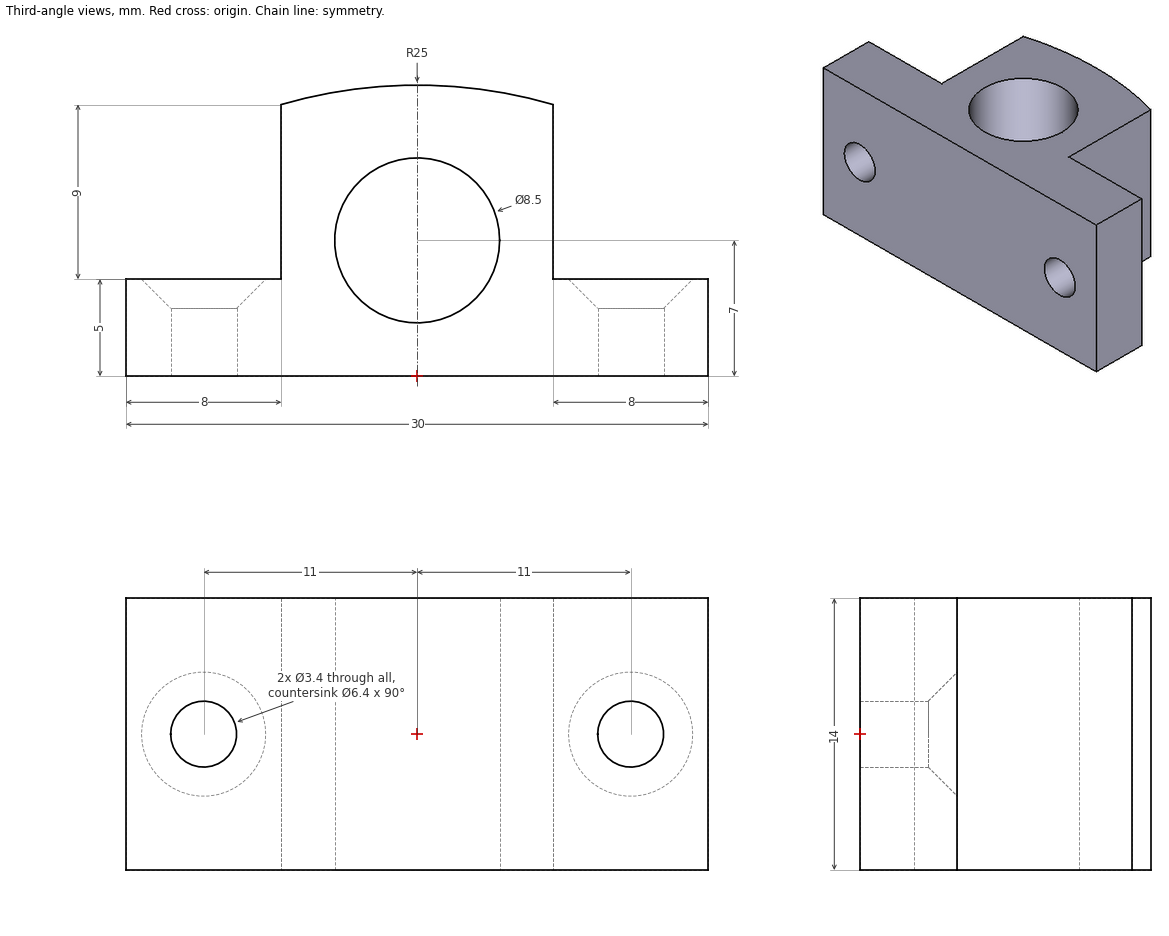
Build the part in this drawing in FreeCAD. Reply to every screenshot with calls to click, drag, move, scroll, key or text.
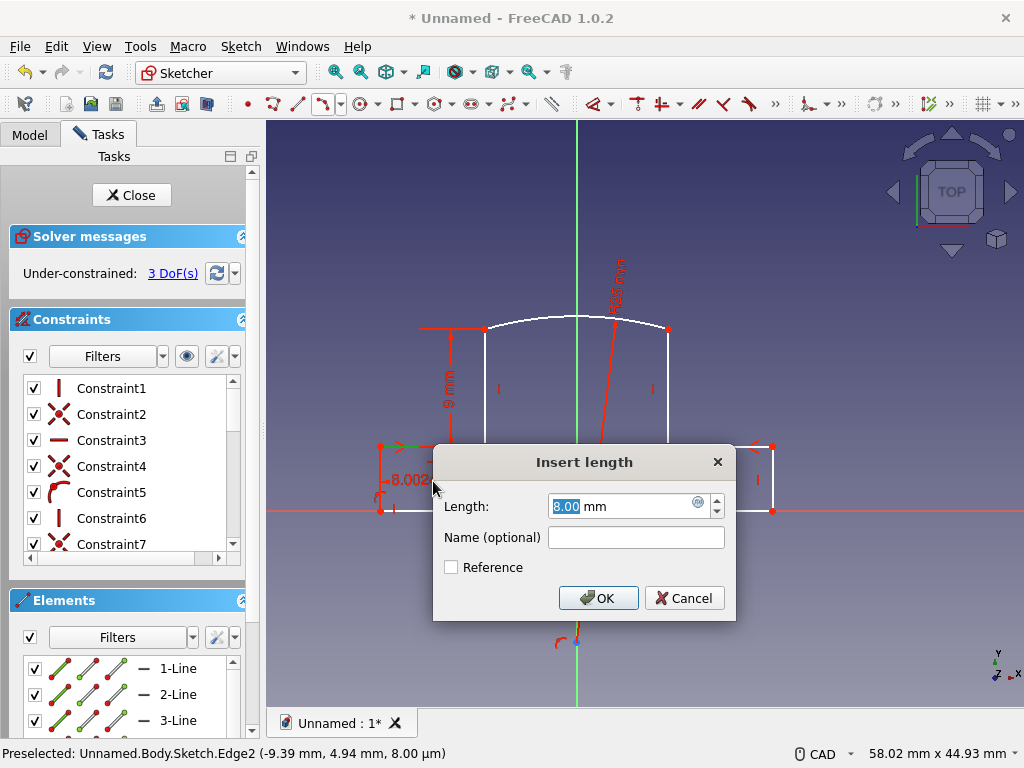
text(8)
key(Return)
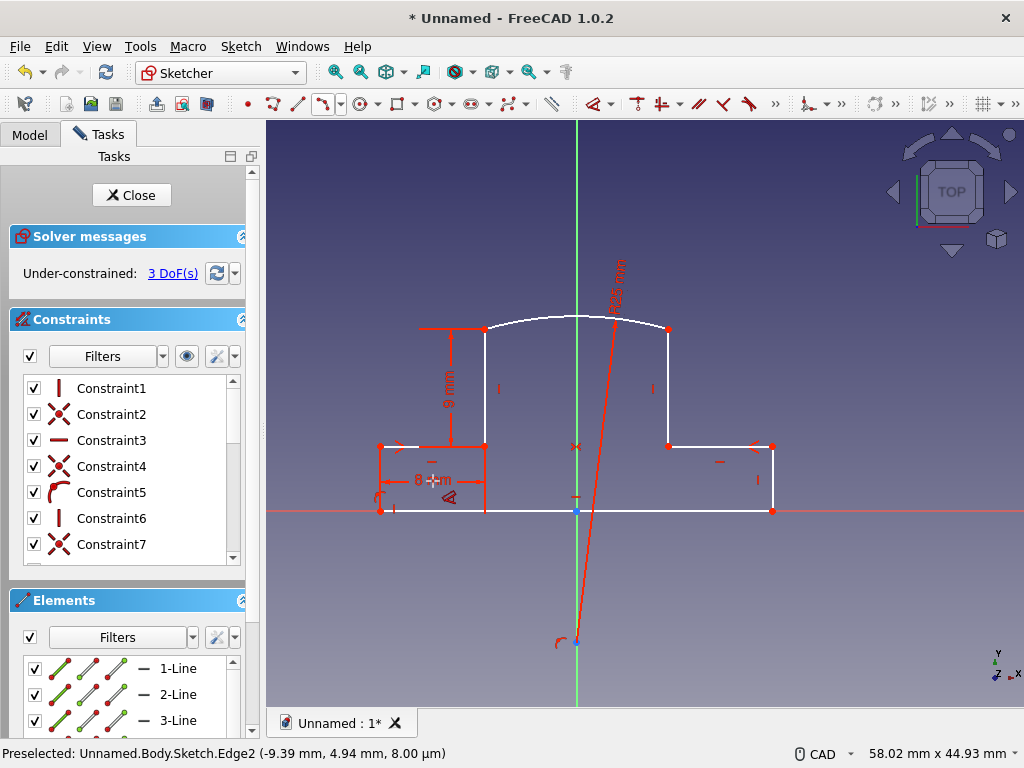
click(380, 466)
click(346, 479)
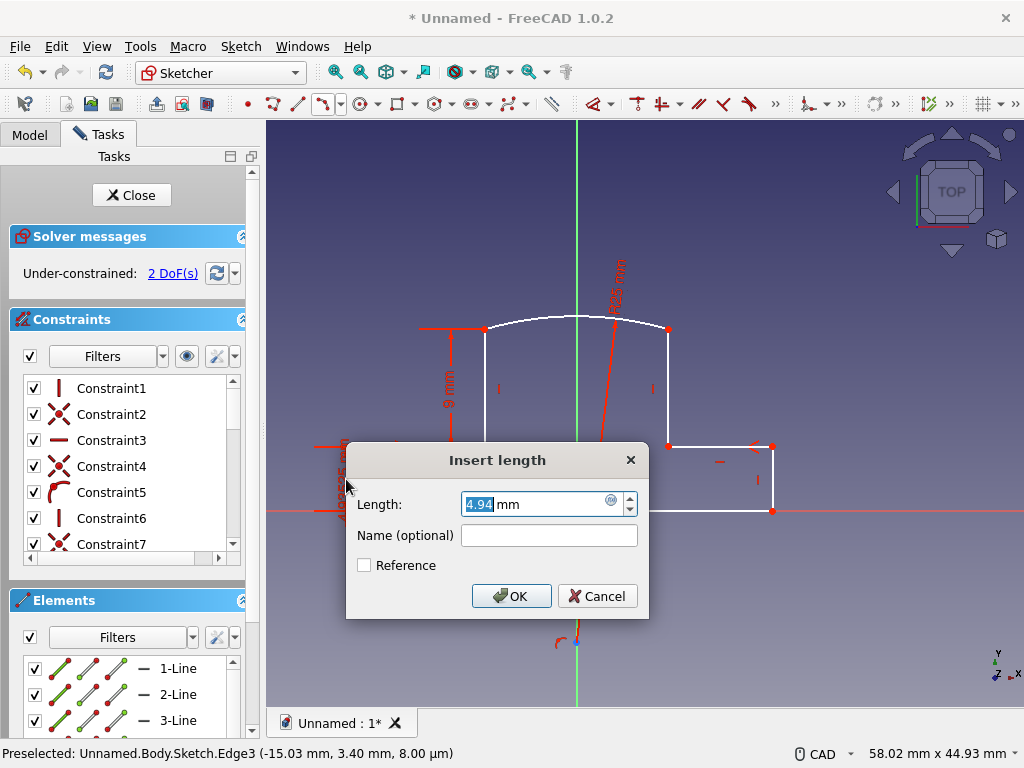
text(5)
key(Return)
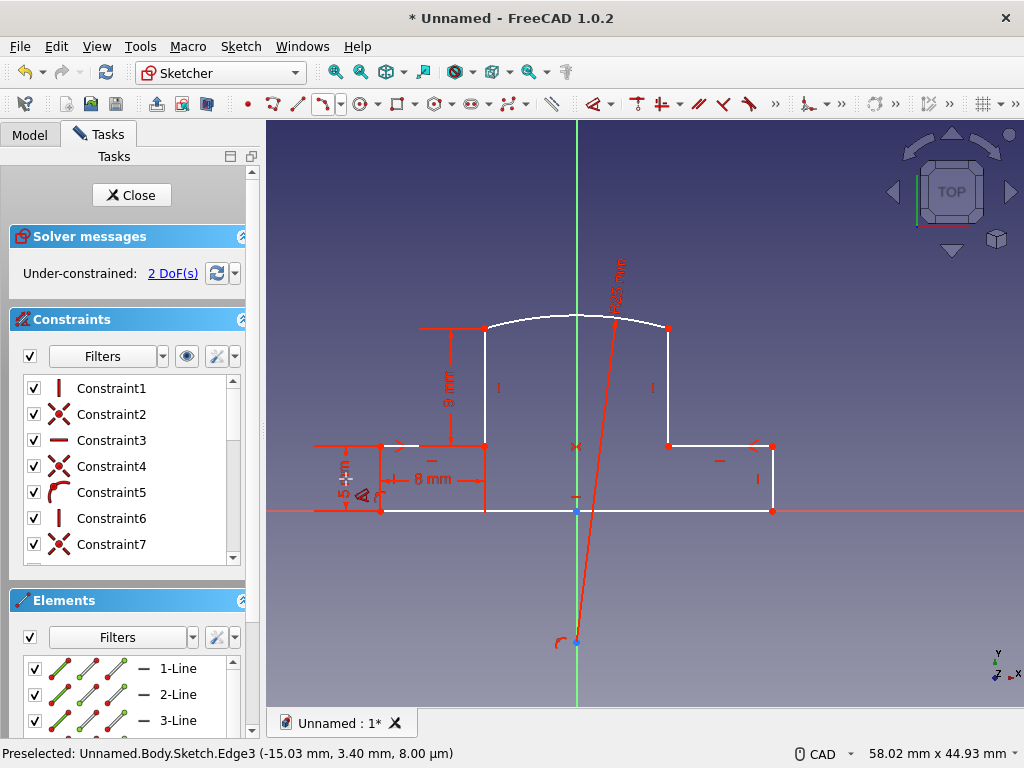
click(742, 446)
click(721, 480)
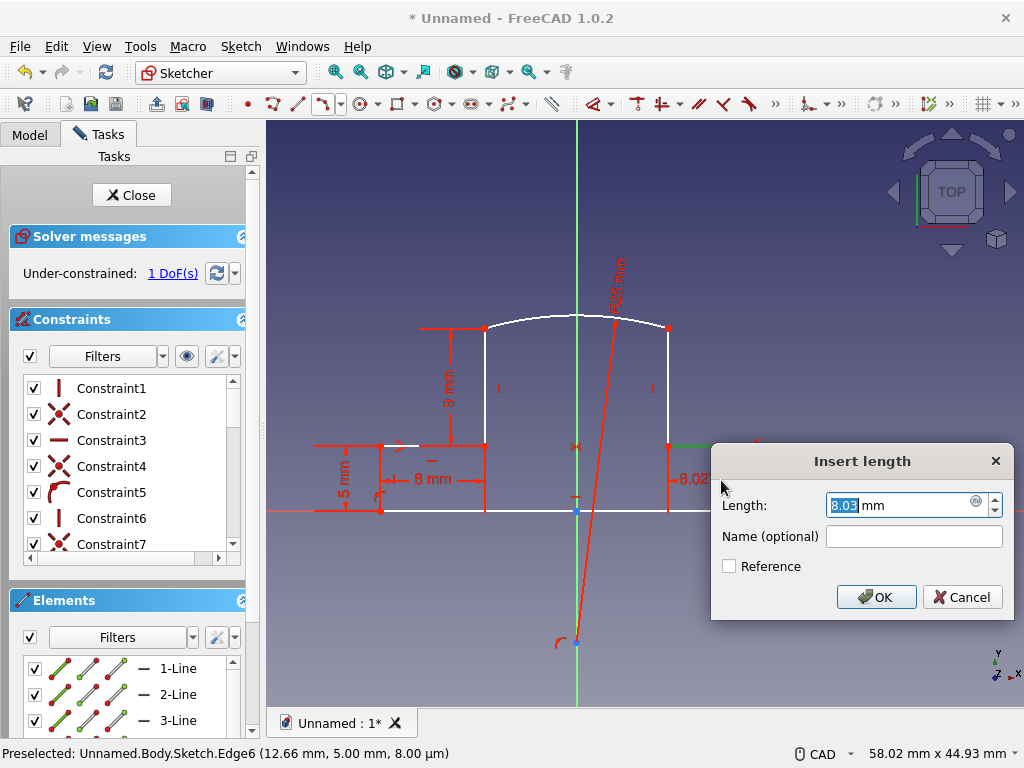
text(8)
key(Return)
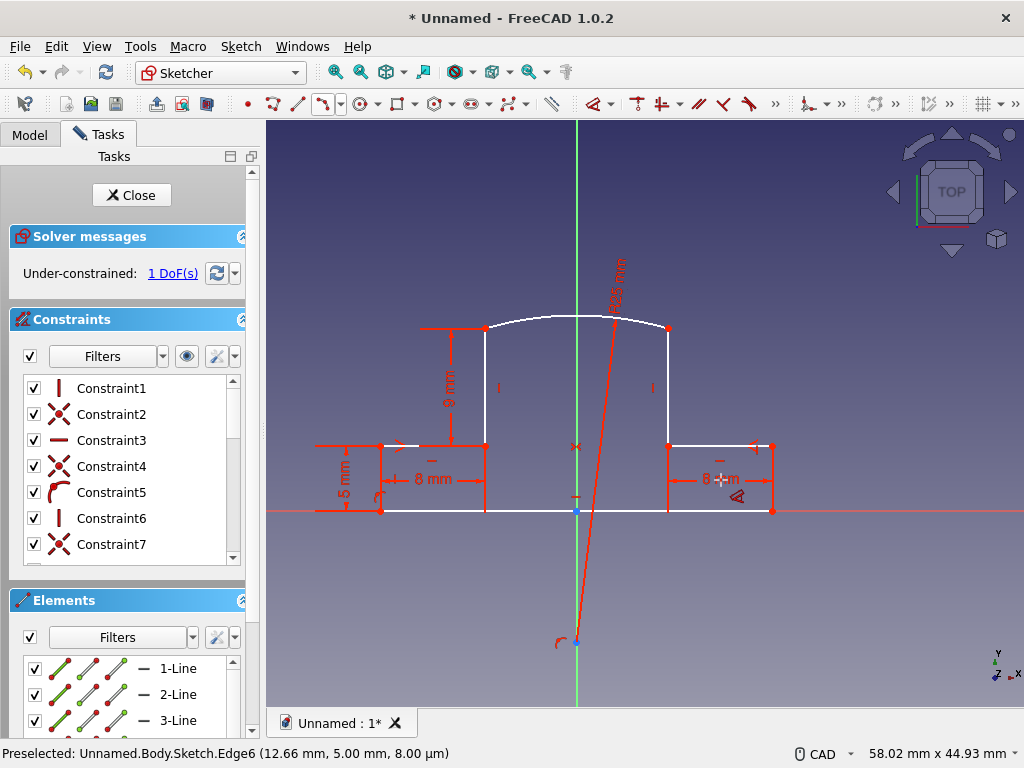
click(498, 511)
click(487, 545)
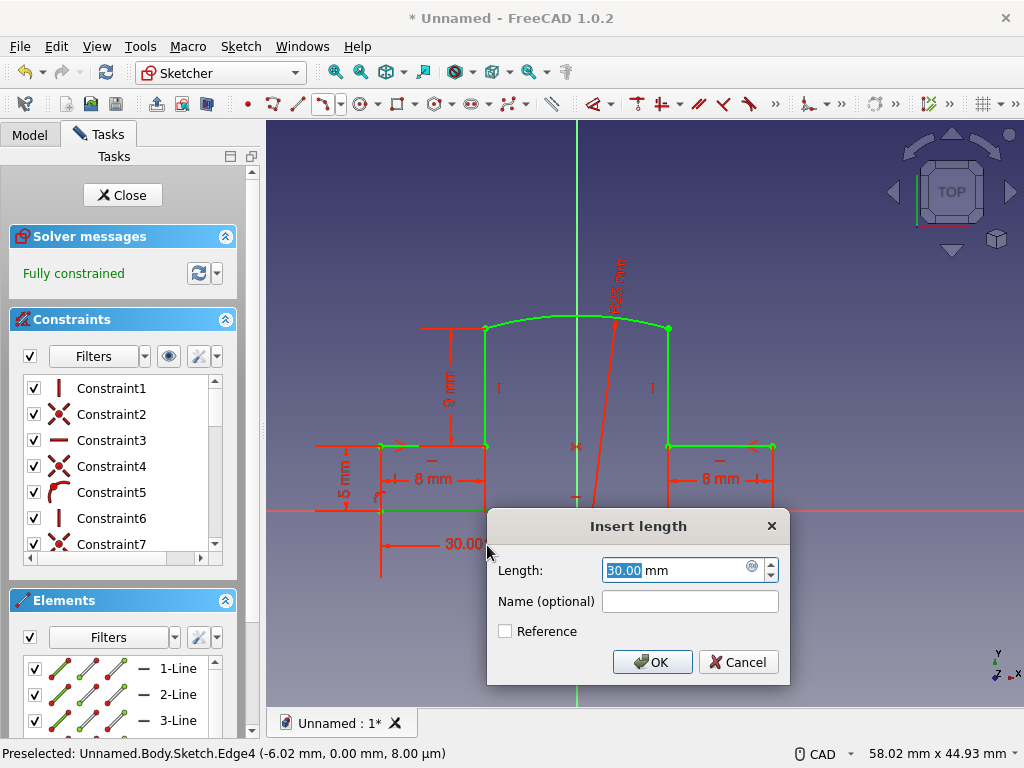
text(30)
key(Return)
key(Escape)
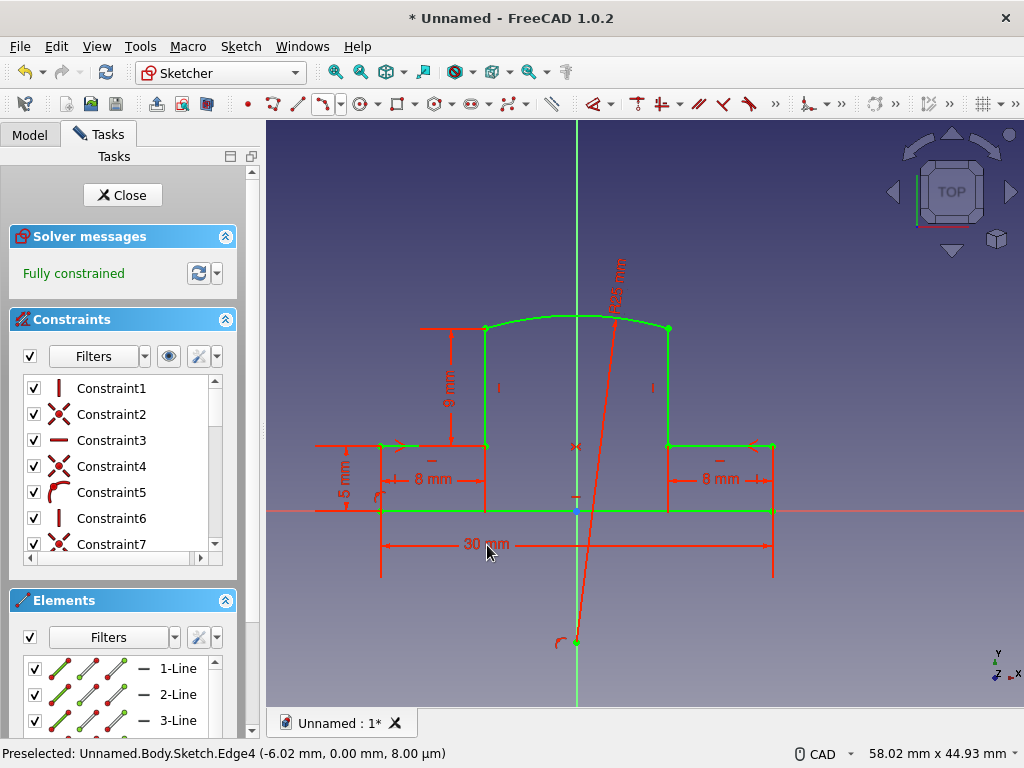
click(123, 195)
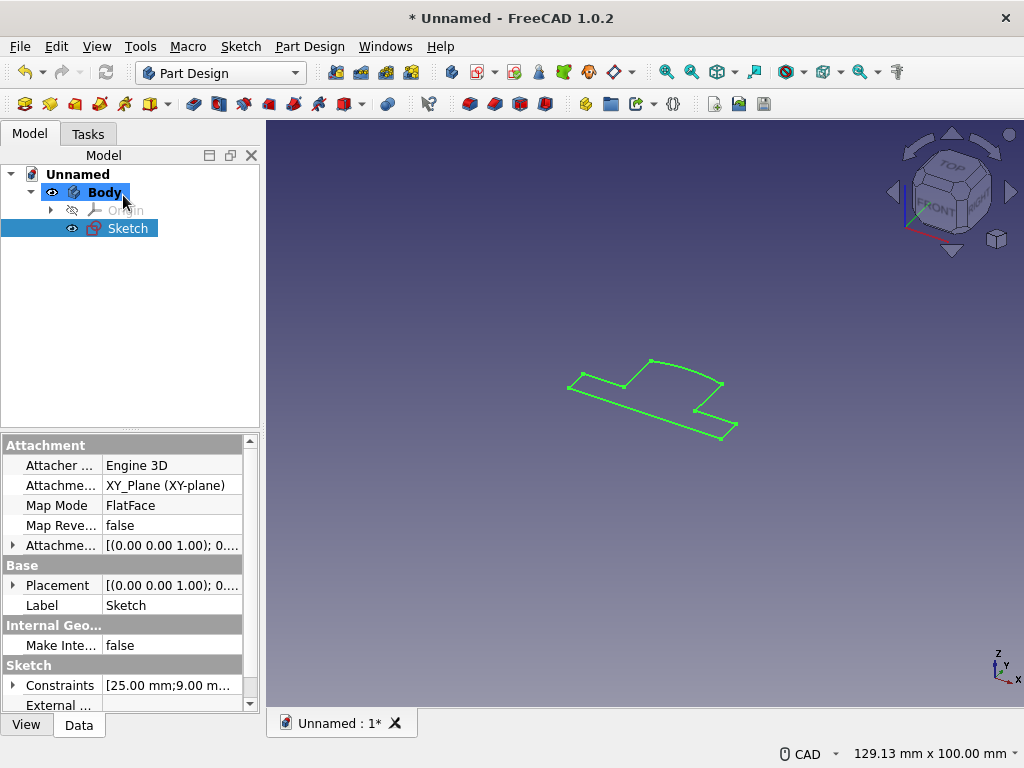
click(25, 104)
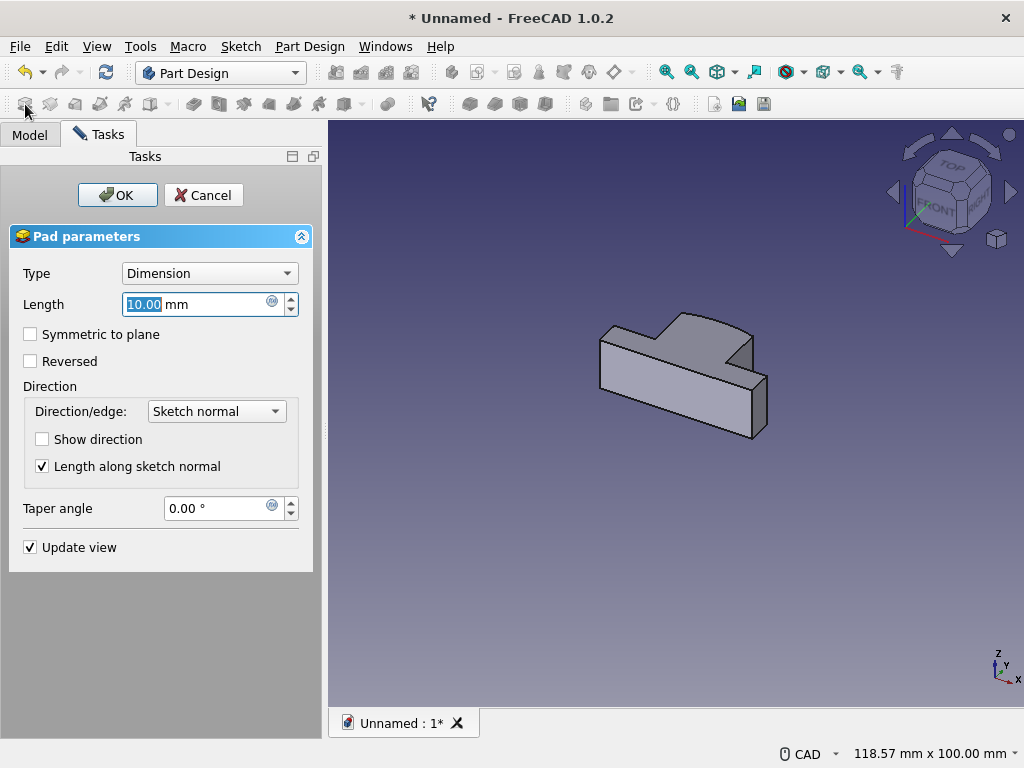
text(14)
key(Tab)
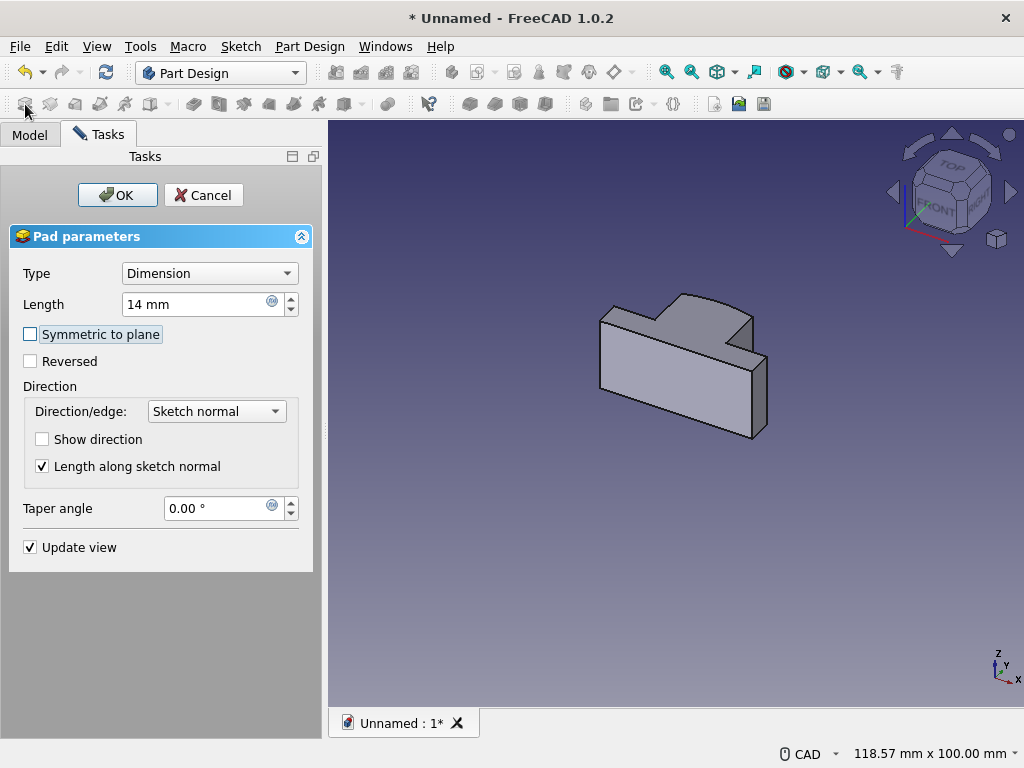
click(31, 334)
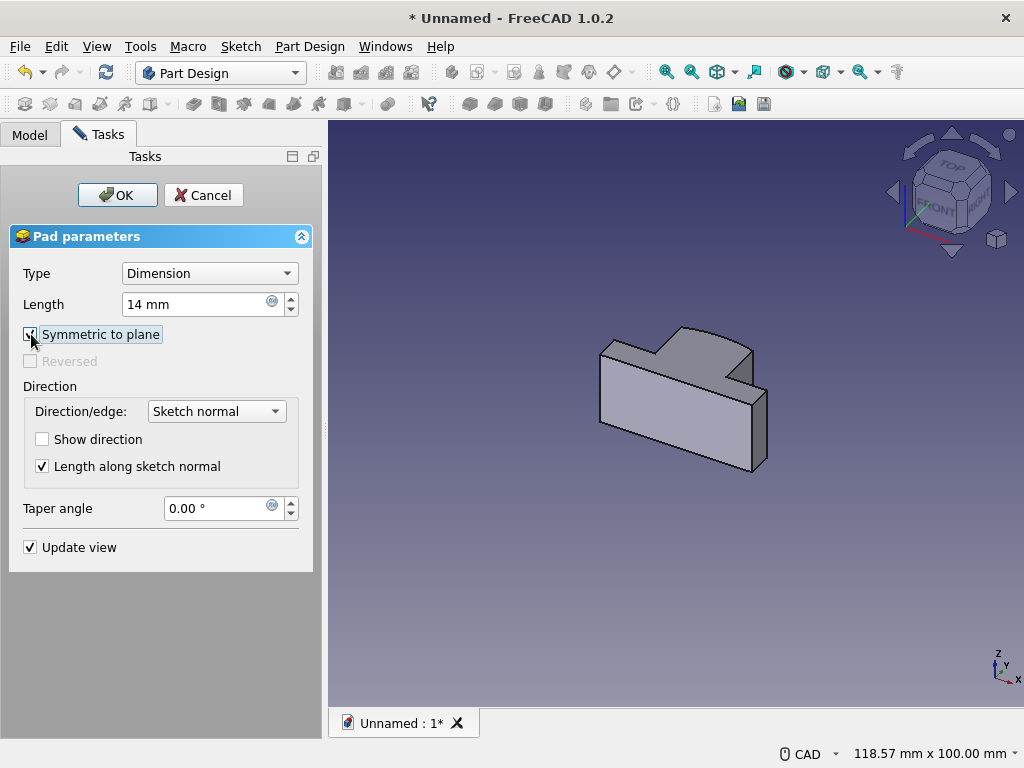
click(118, 195)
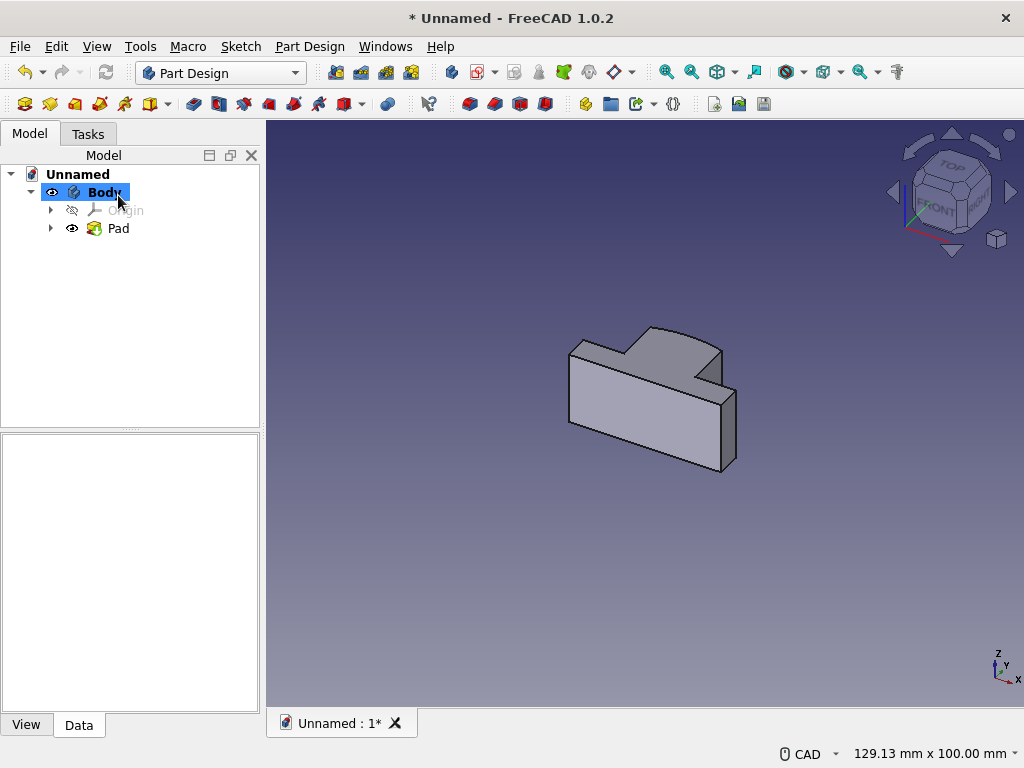
click(667, 72)